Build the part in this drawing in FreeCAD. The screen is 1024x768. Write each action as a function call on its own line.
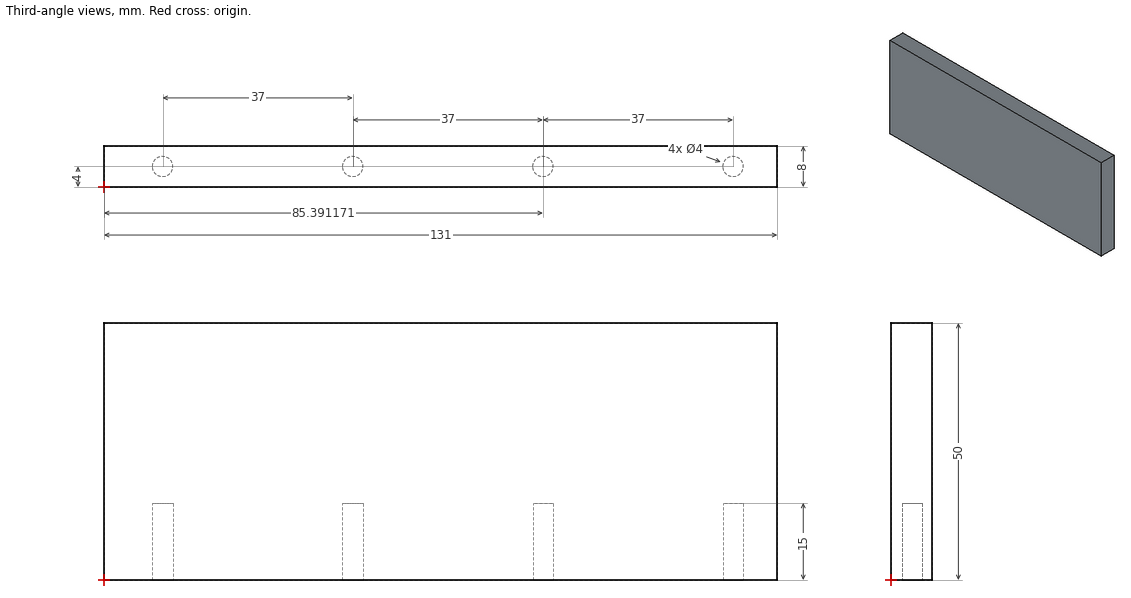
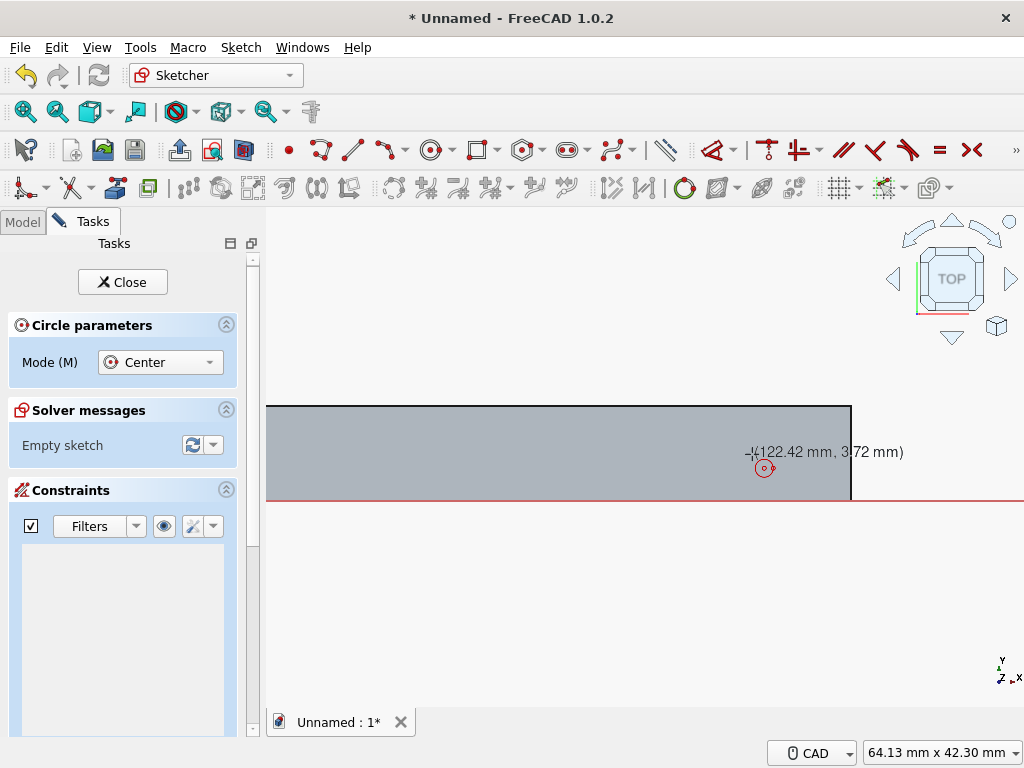
scroll(753, 454, down, 7)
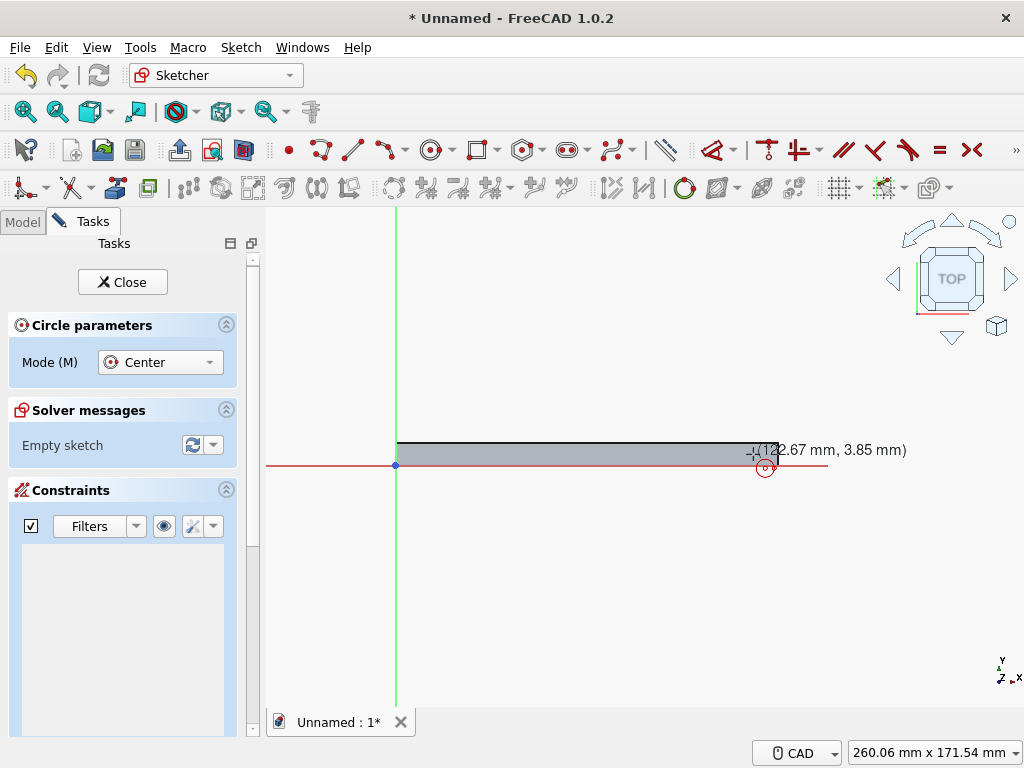
scroll(753, 454, up, 2)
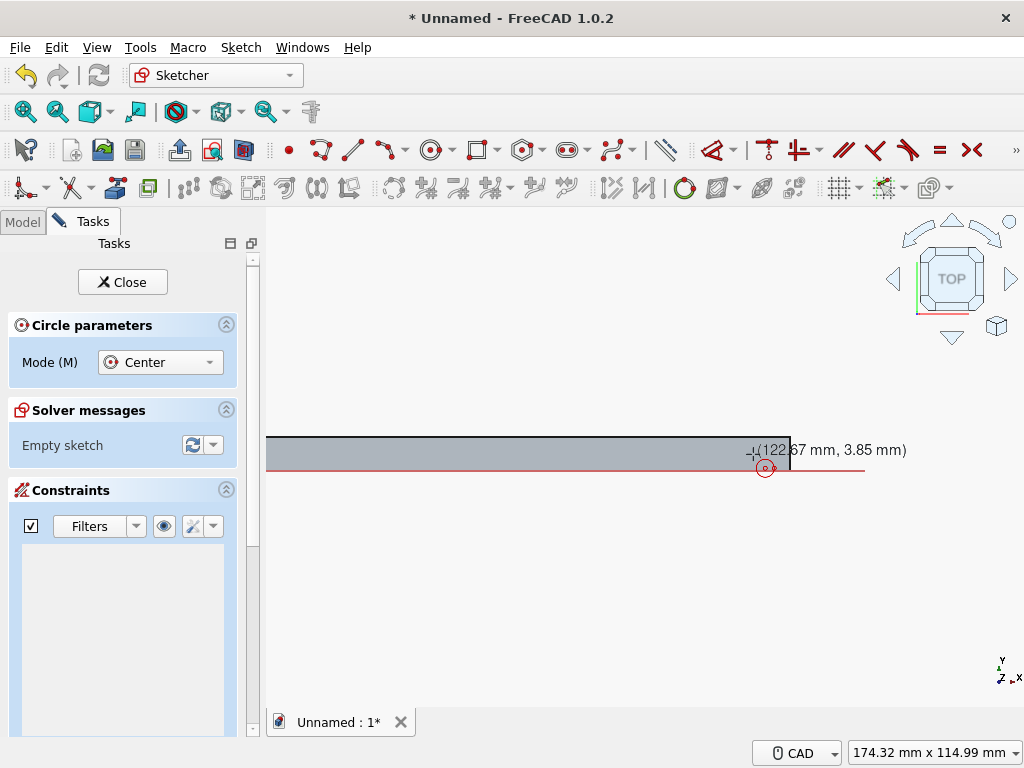
click(752, 454)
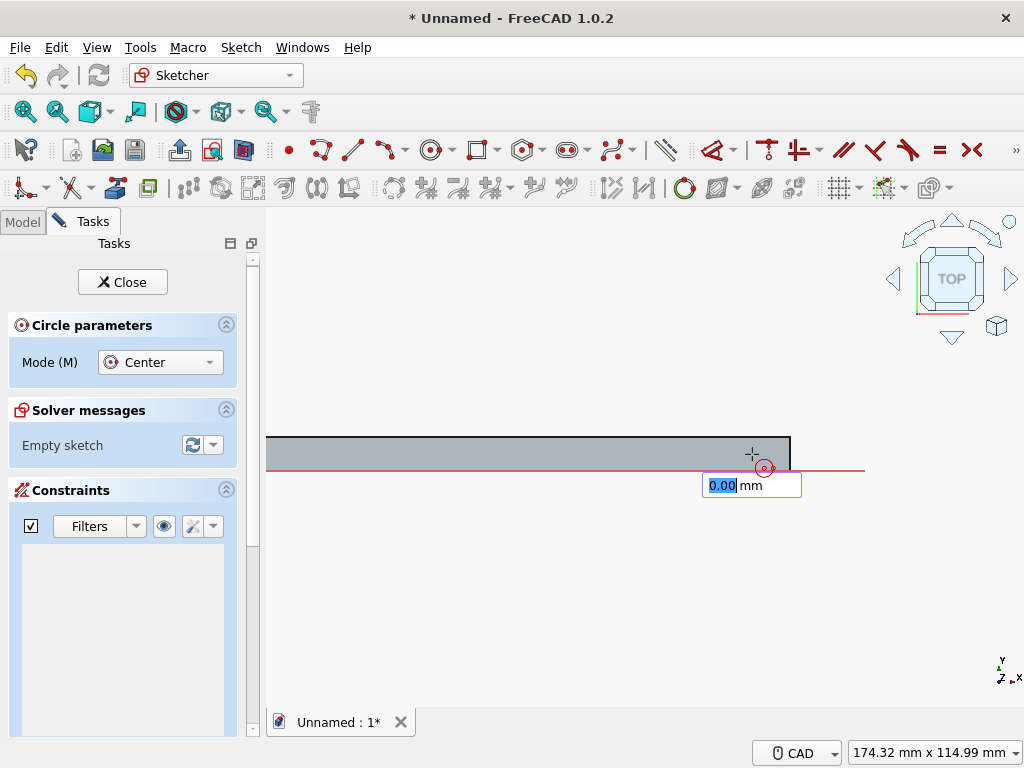
scroll(758, 448, up, 4)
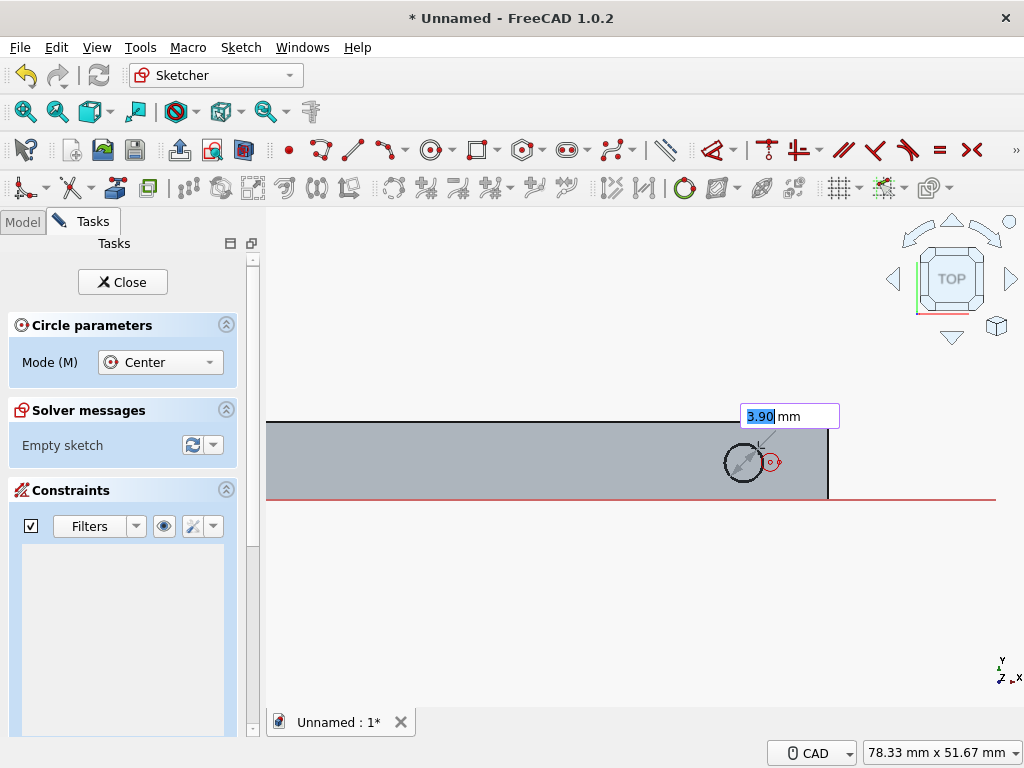
click(758, 447)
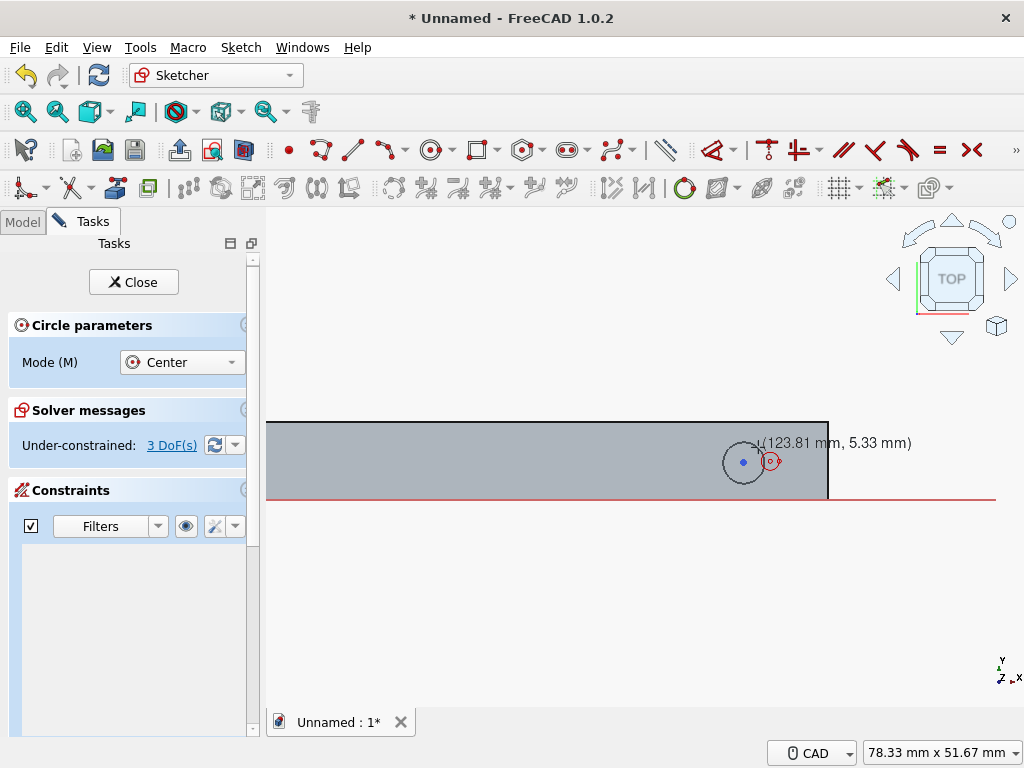
click(386, 461)
click(400, 447)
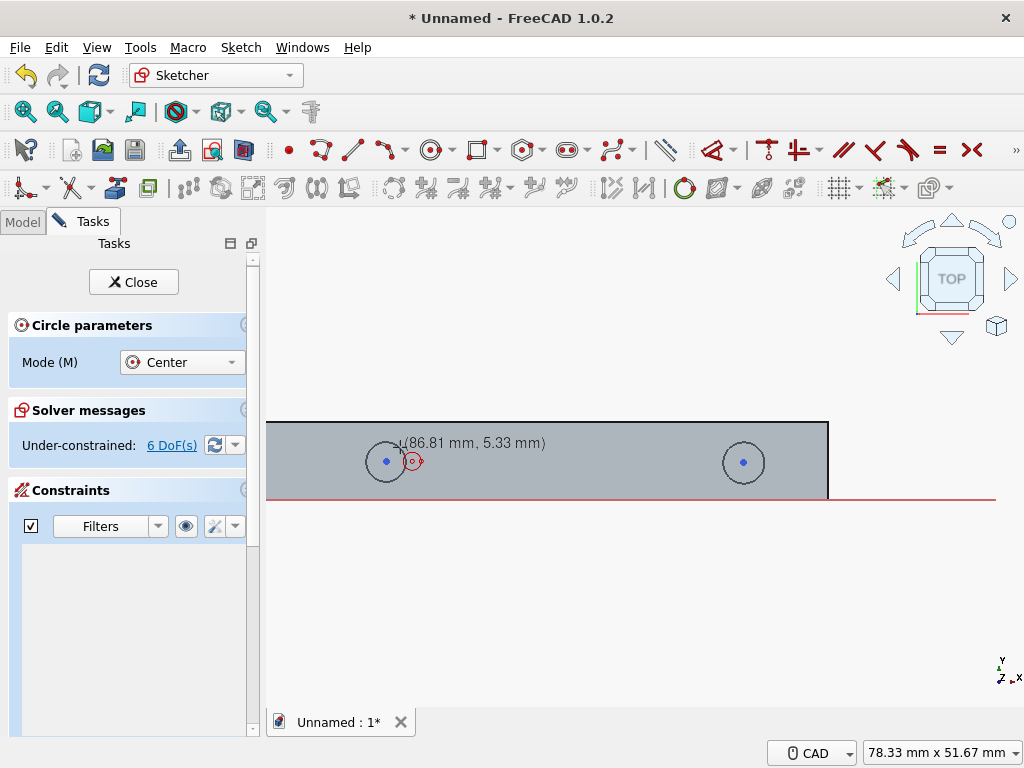
scroll(755, 451, down, 6)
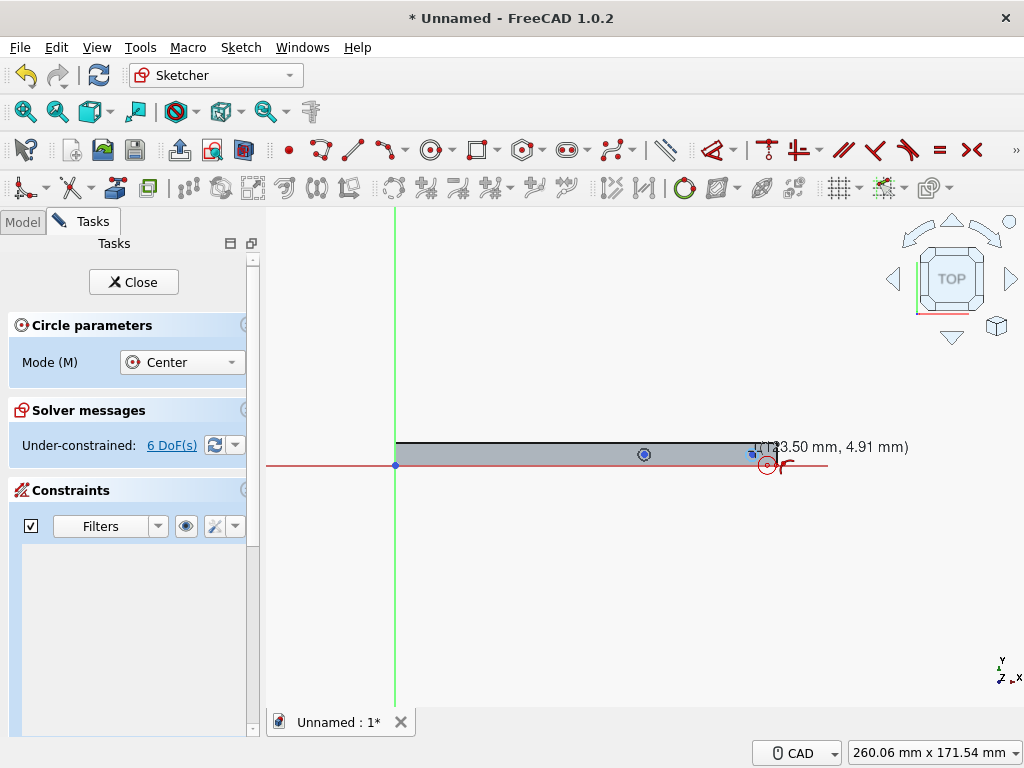
scroll(537, 454, up, 7)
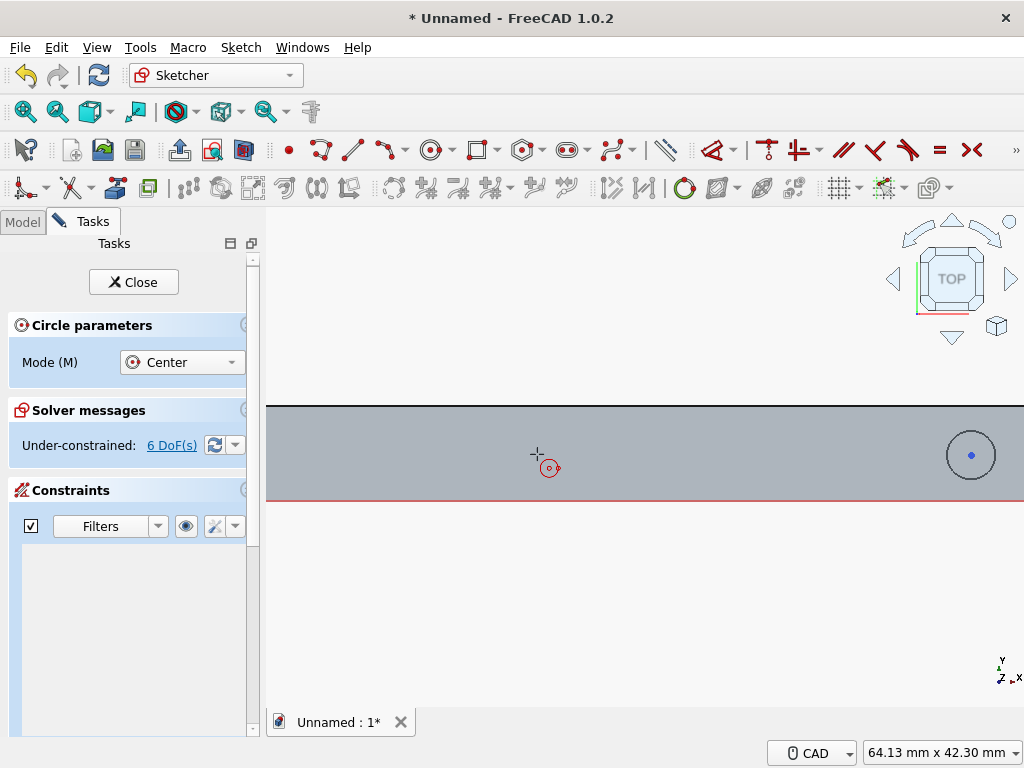
scroll(537, 454, down, 7)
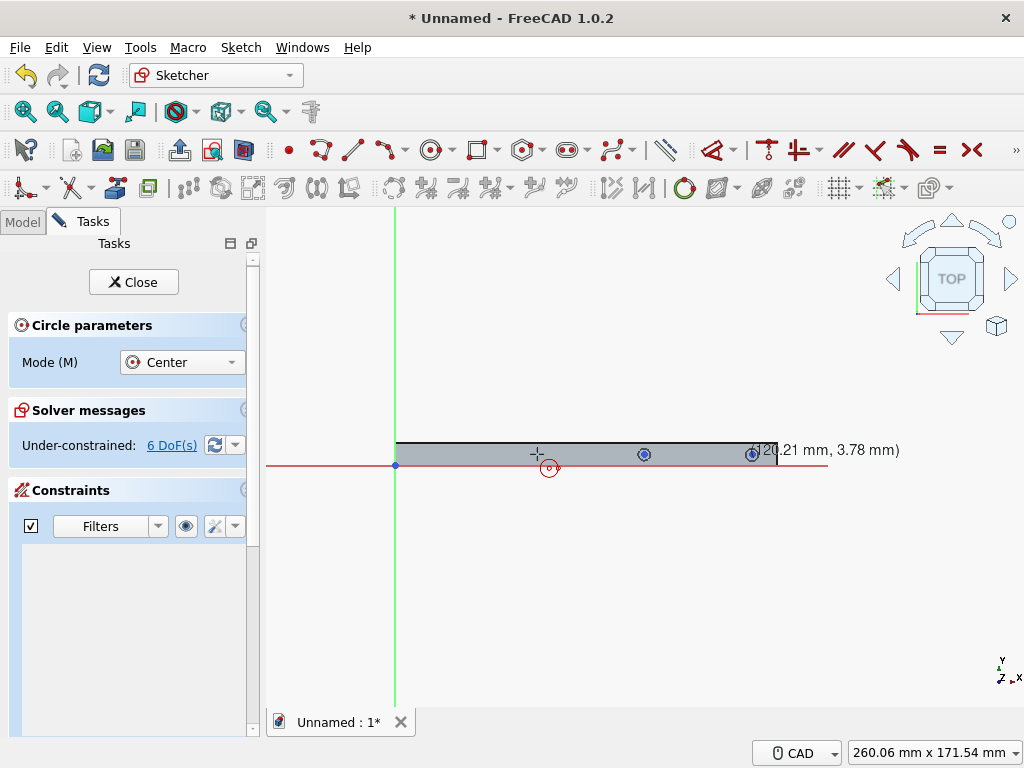
scroll(537, 454, up, 2)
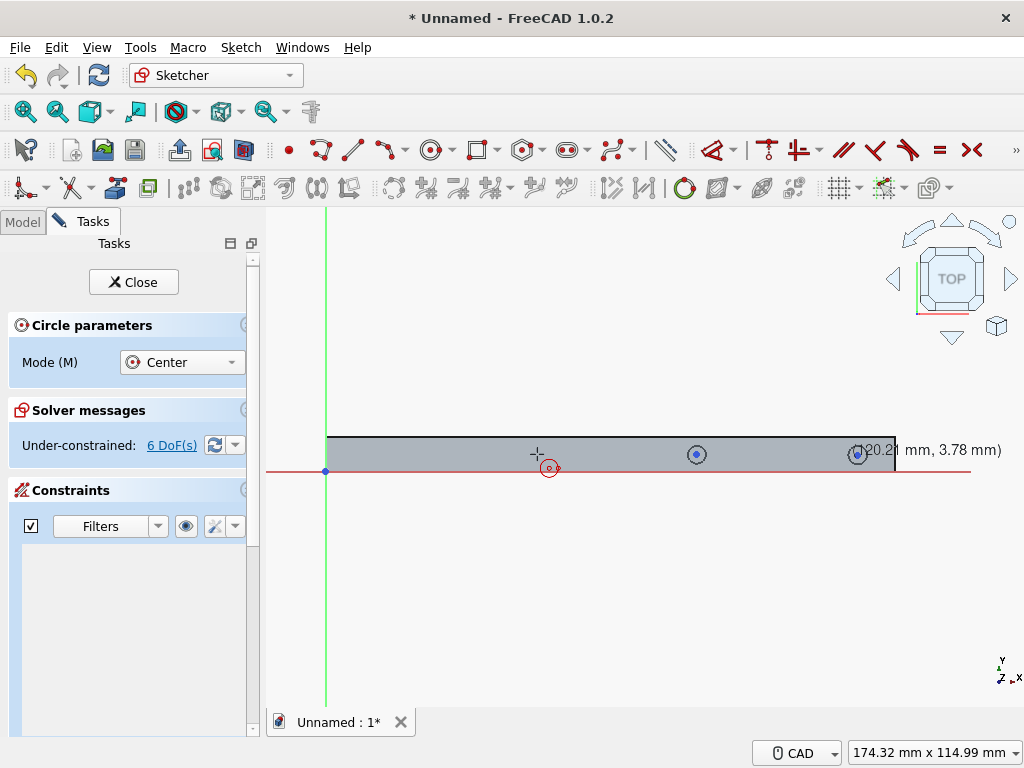
click(536, 454)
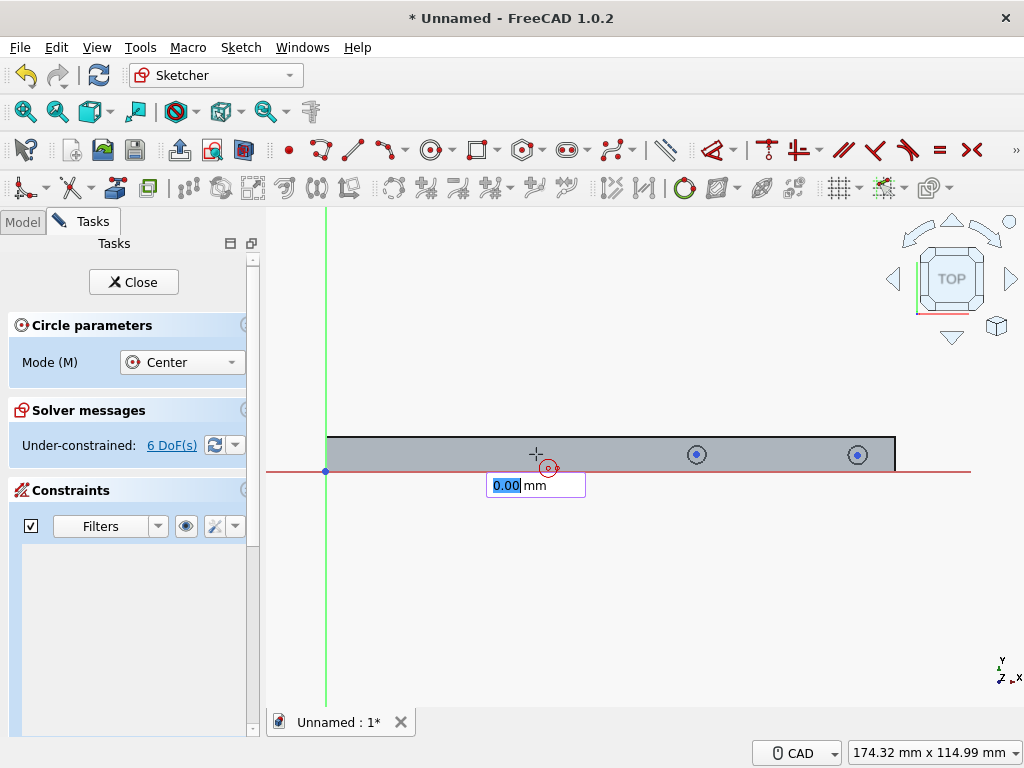
scroll(542, 448, up, 4)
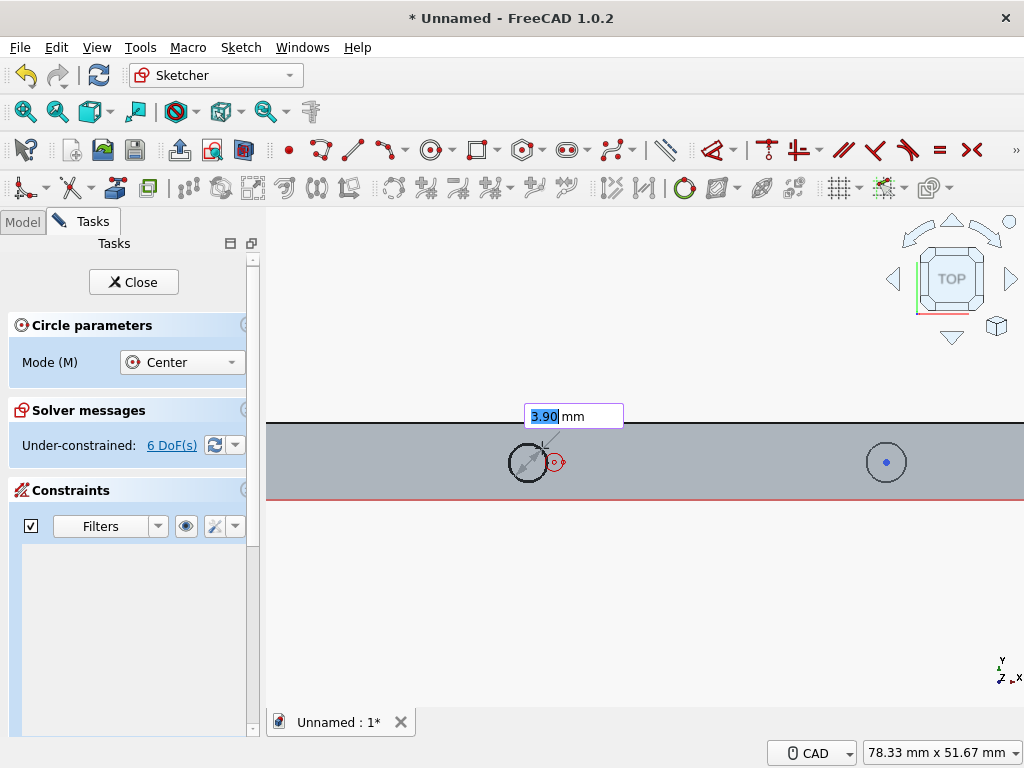
click(542, 448)